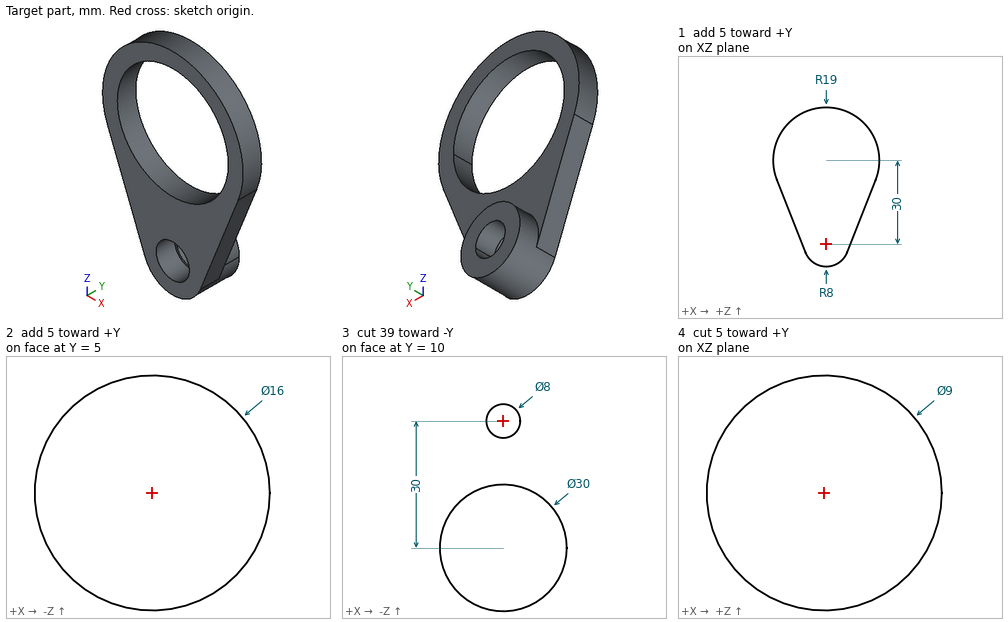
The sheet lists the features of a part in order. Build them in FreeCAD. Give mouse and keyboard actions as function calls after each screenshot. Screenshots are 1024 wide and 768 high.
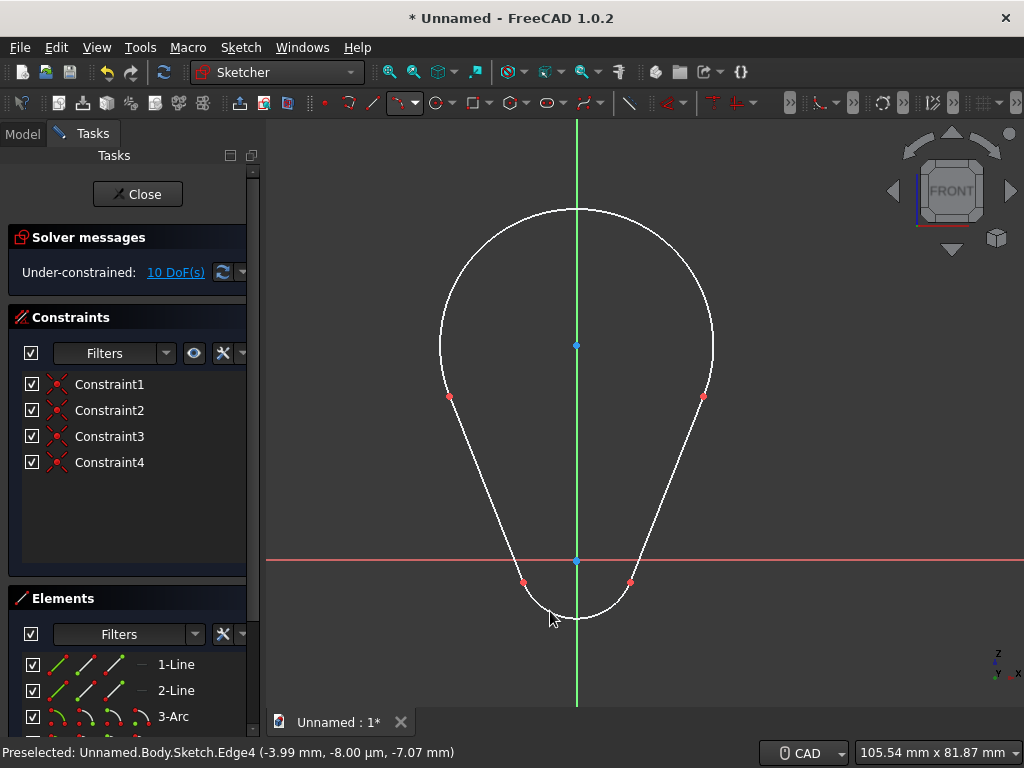
click(501, 527)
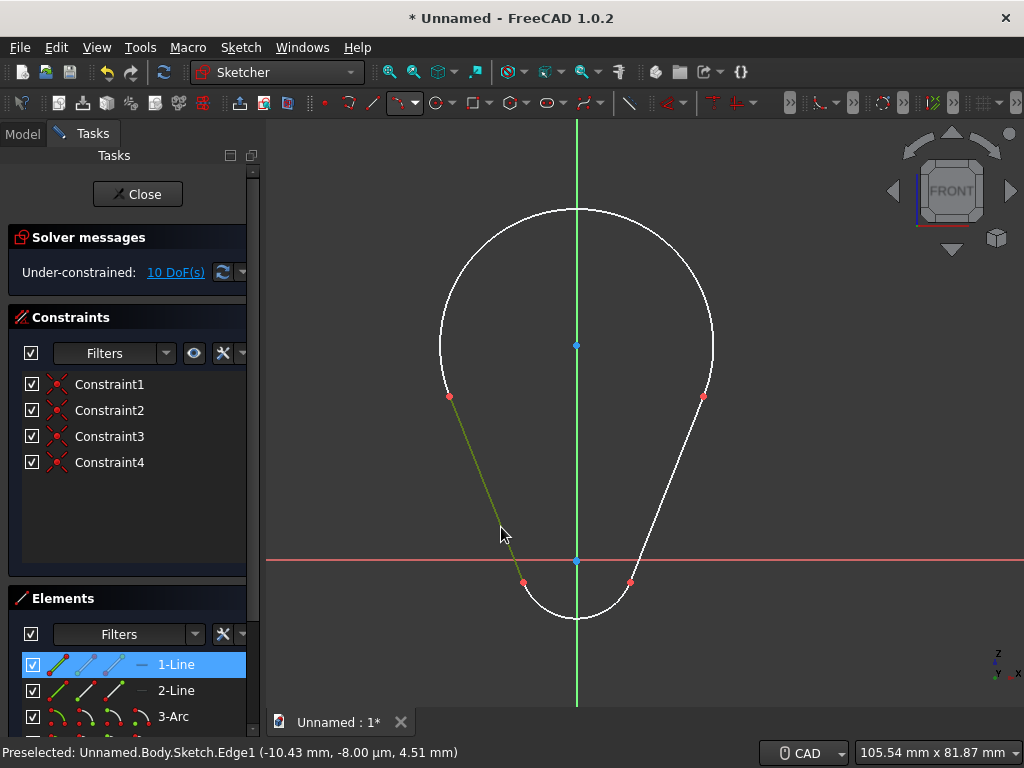
click(673, 248)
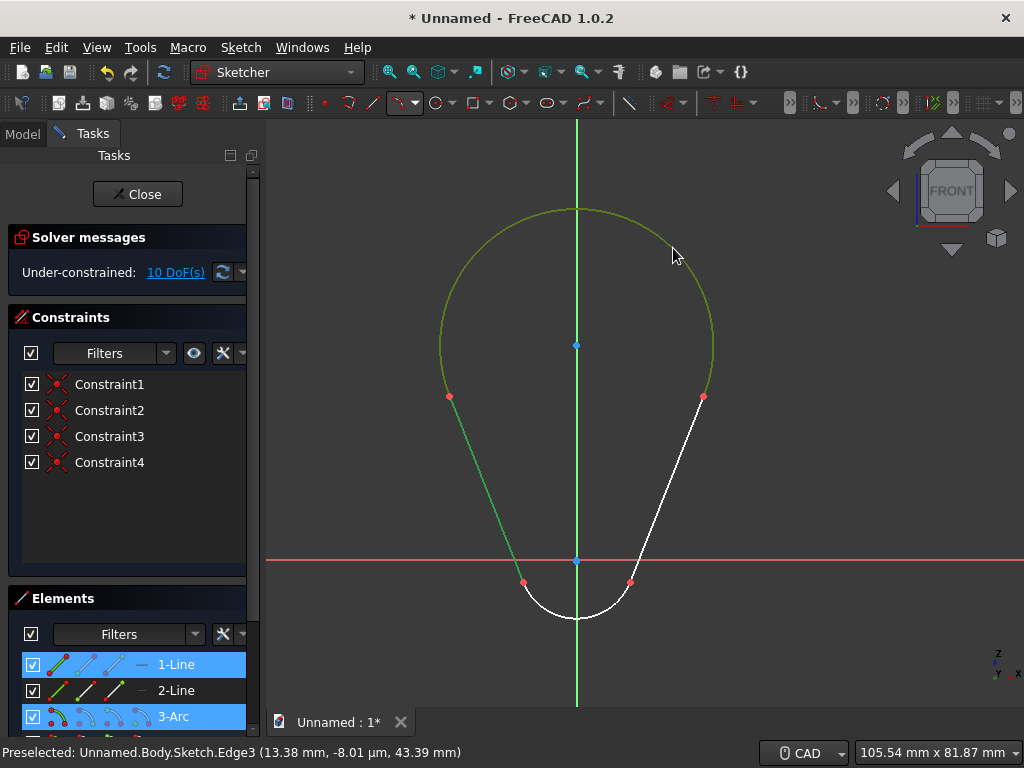
key(t)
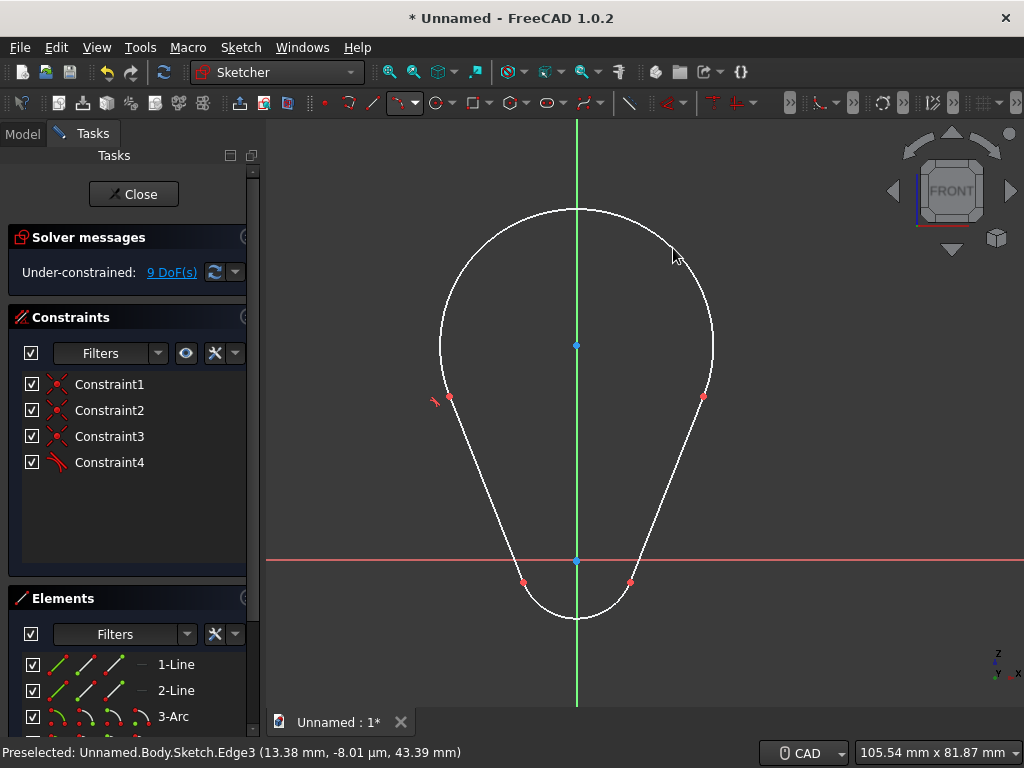
click(501, 527)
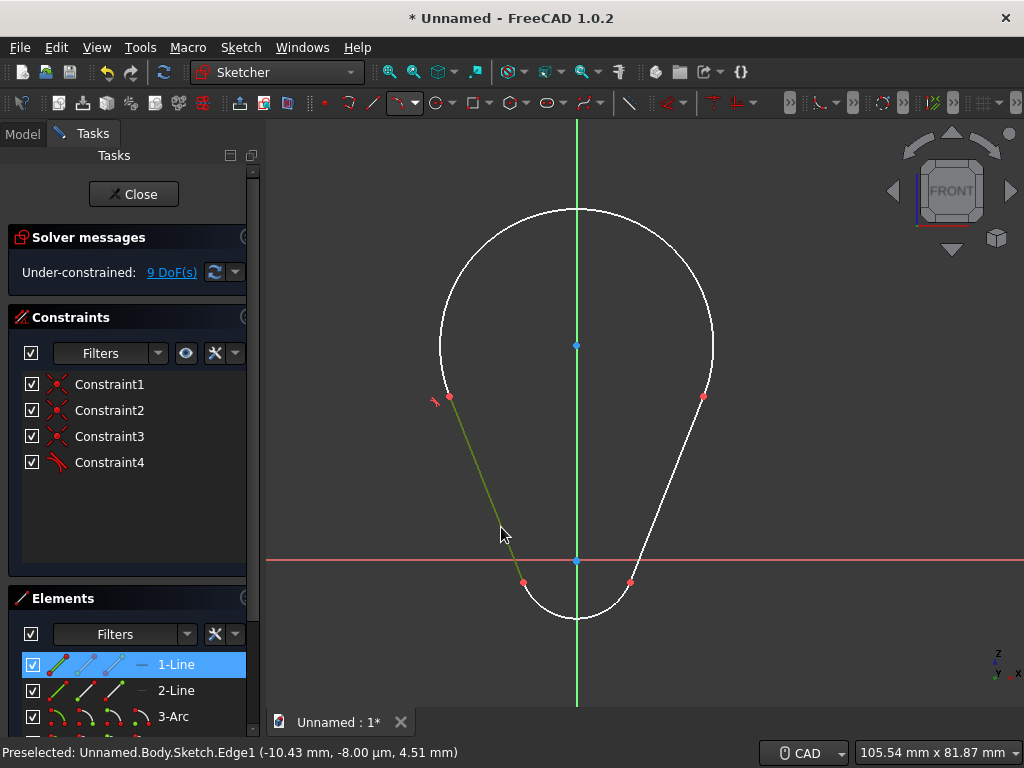
click(550, 612)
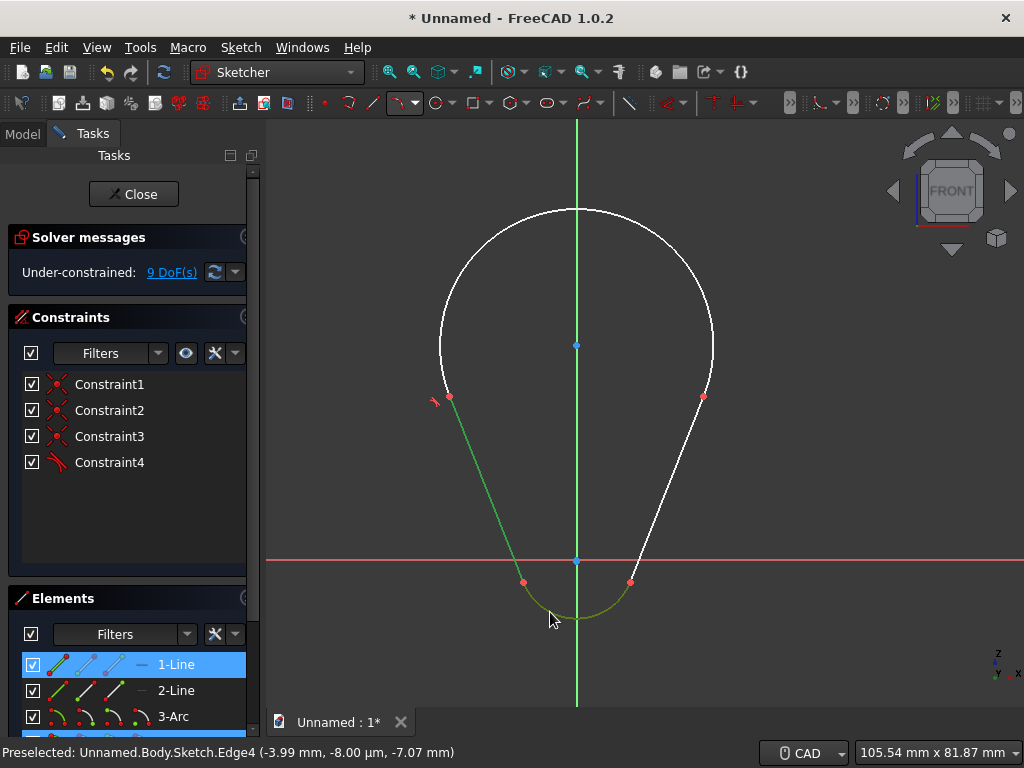
key(t)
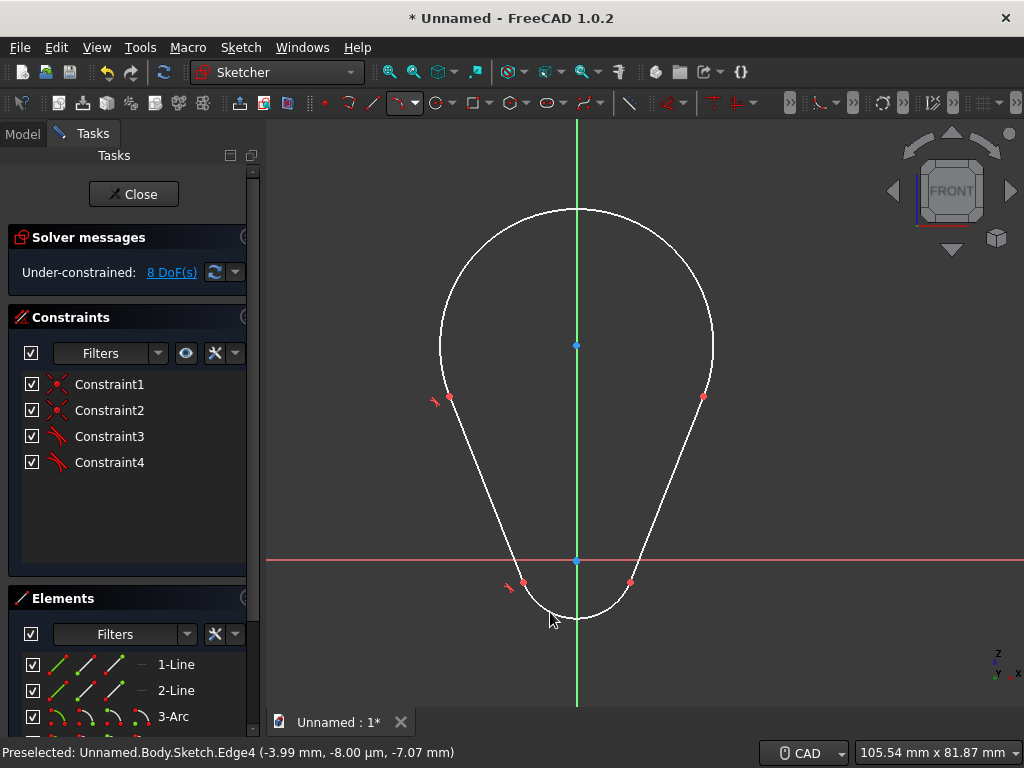
click(682, 452)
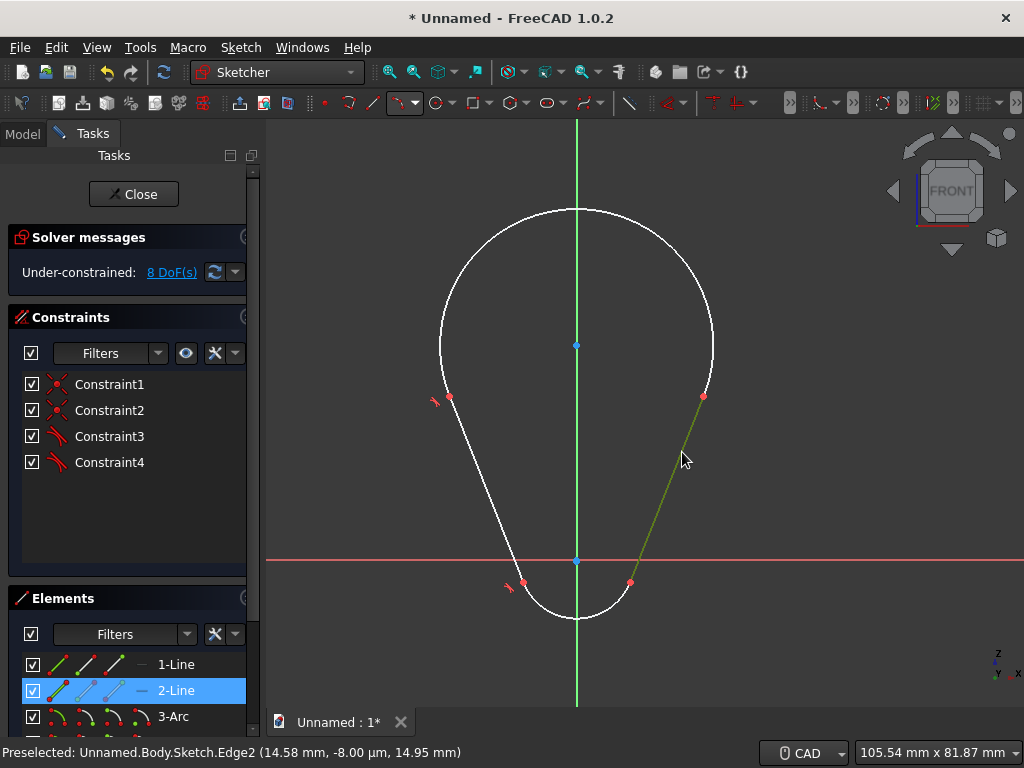
click(673, 249)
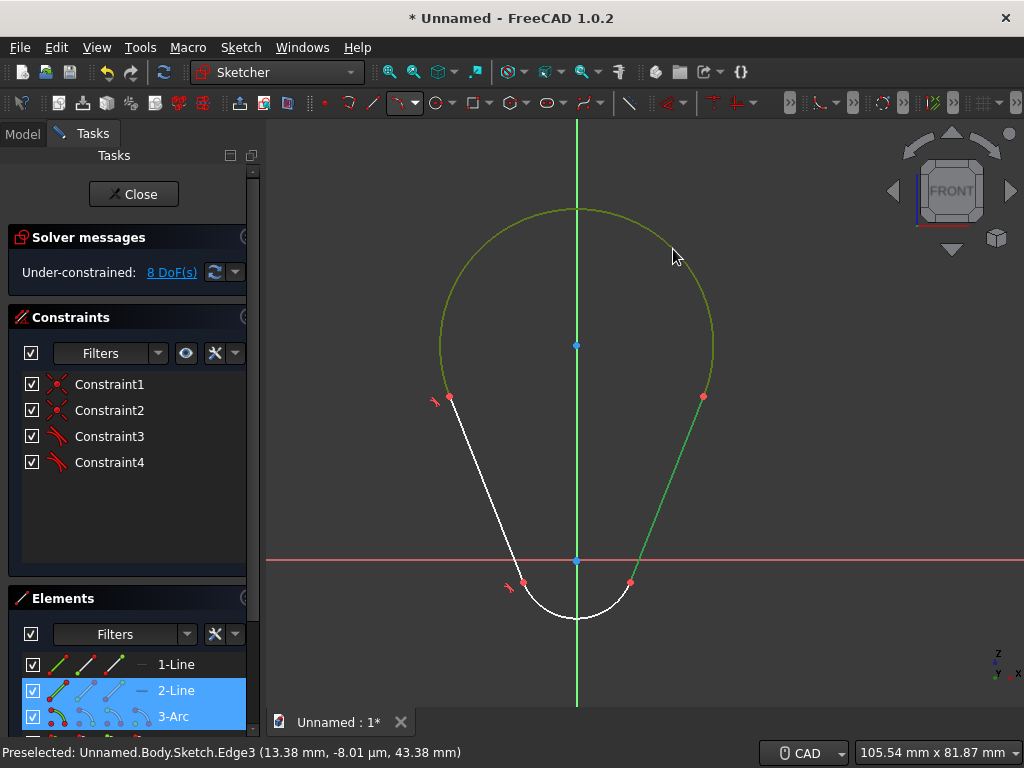
key(t)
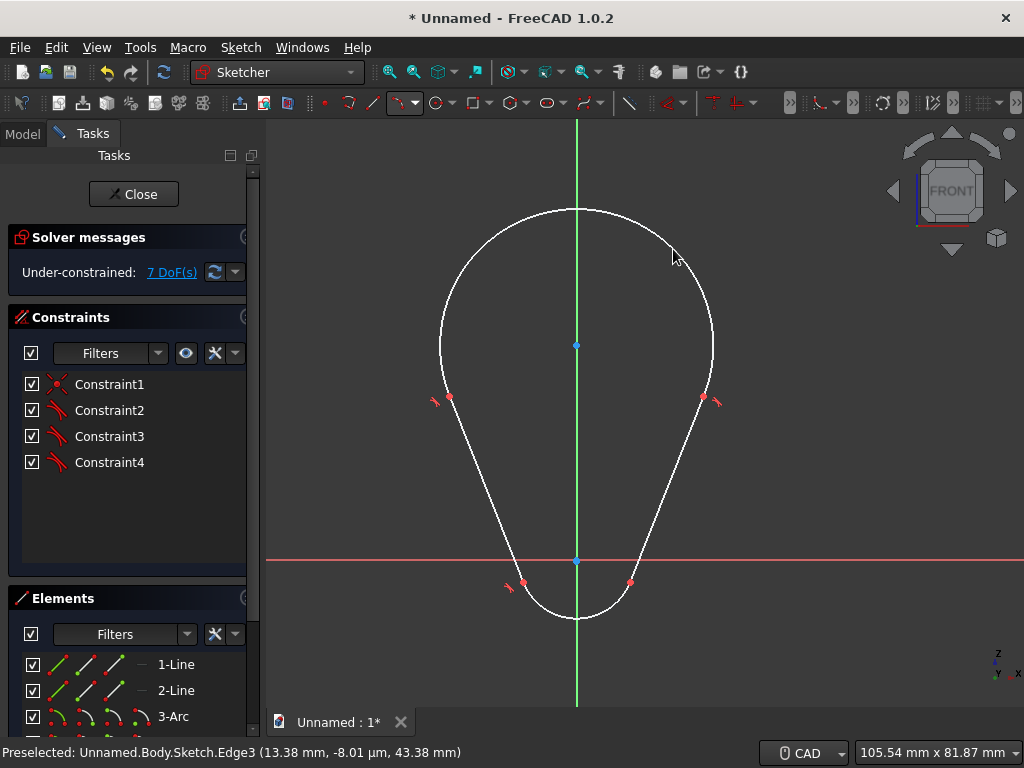
click(682, 452)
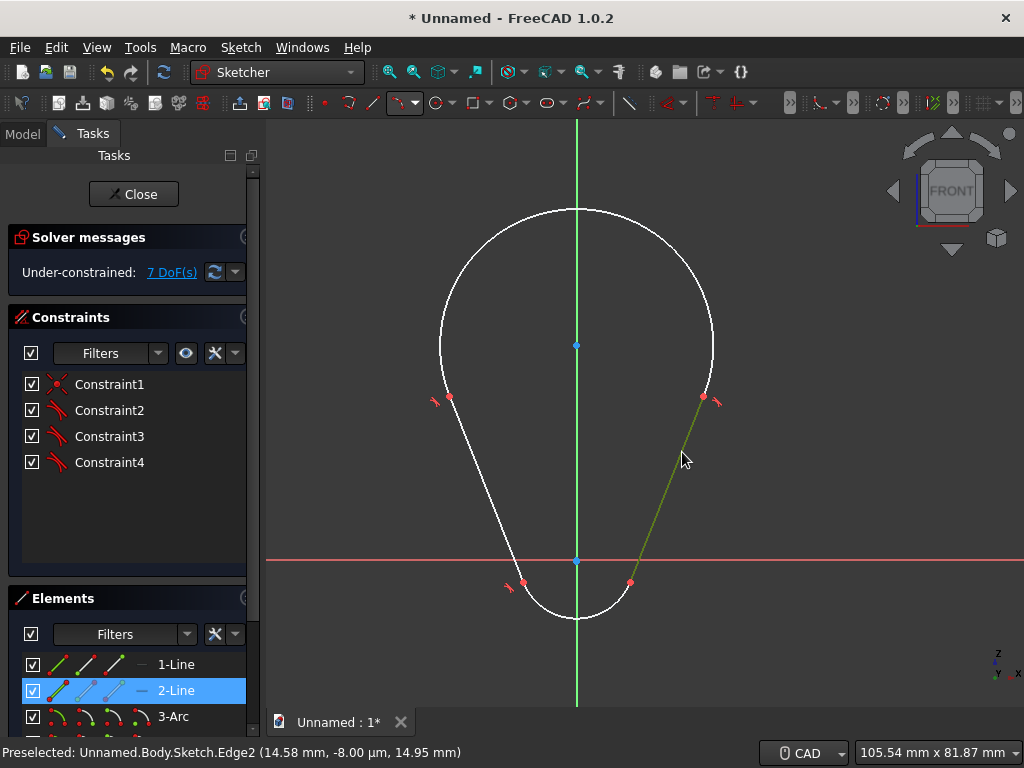
click(550, 612)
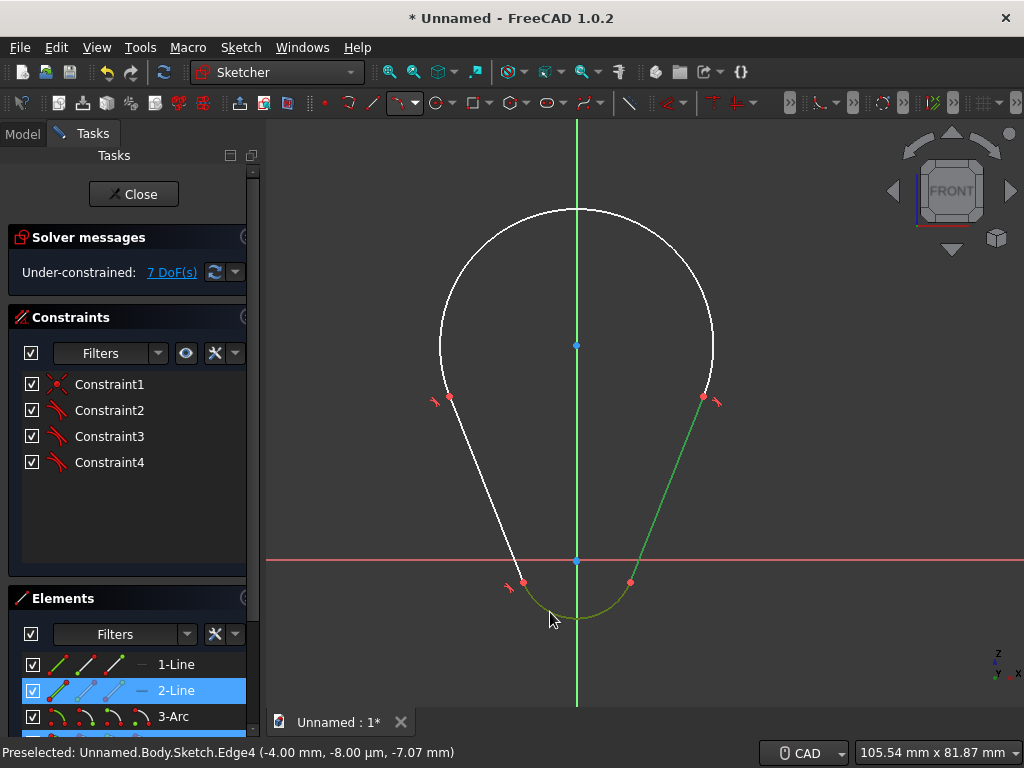
key(t)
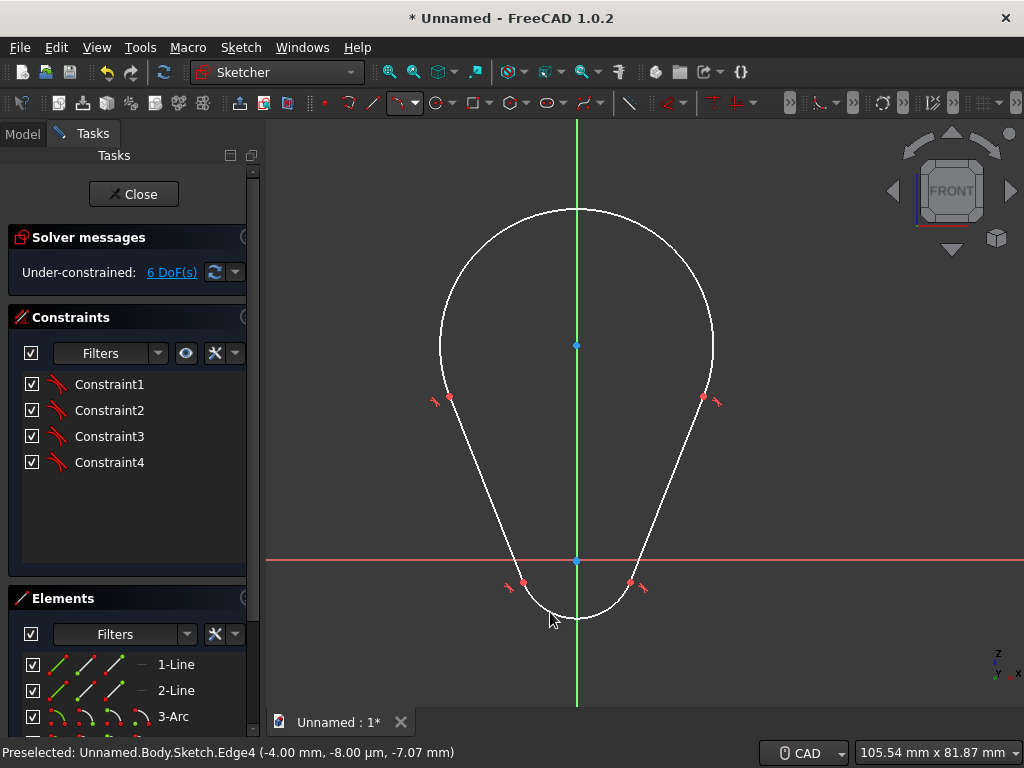
drag(567, 550, 587, 571)